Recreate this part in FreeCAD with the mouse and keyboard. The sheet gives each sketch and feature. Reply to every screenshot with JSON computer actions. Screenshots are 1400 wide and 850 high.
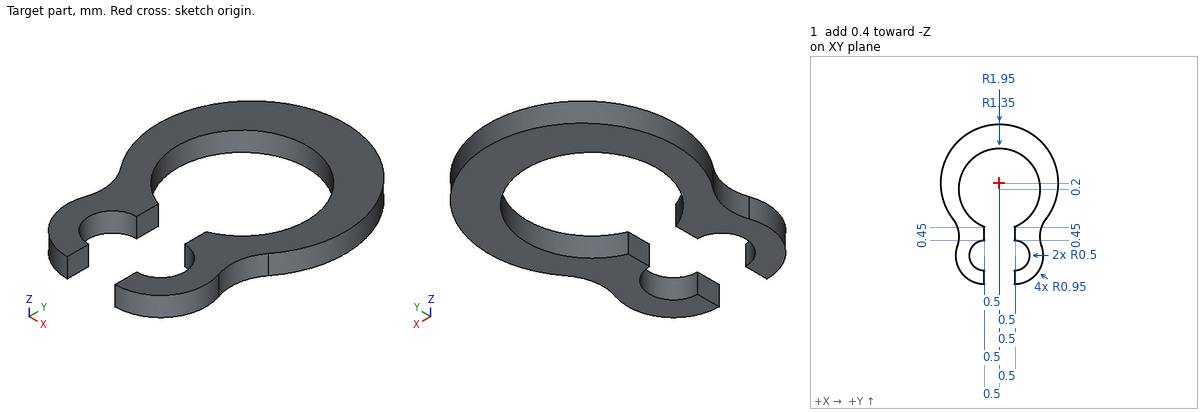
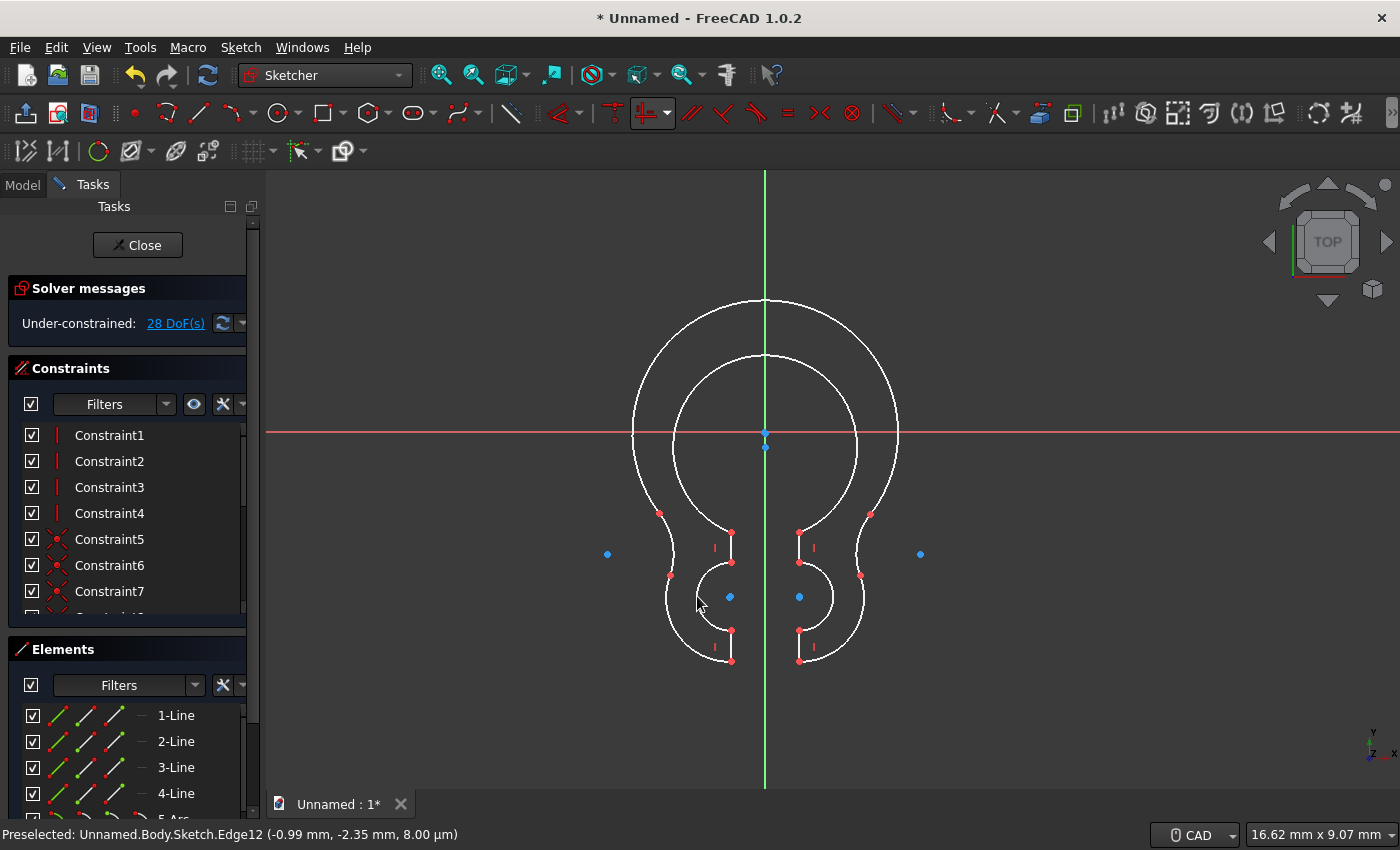
{"action": "left_click", "coordinate": [834, 652]}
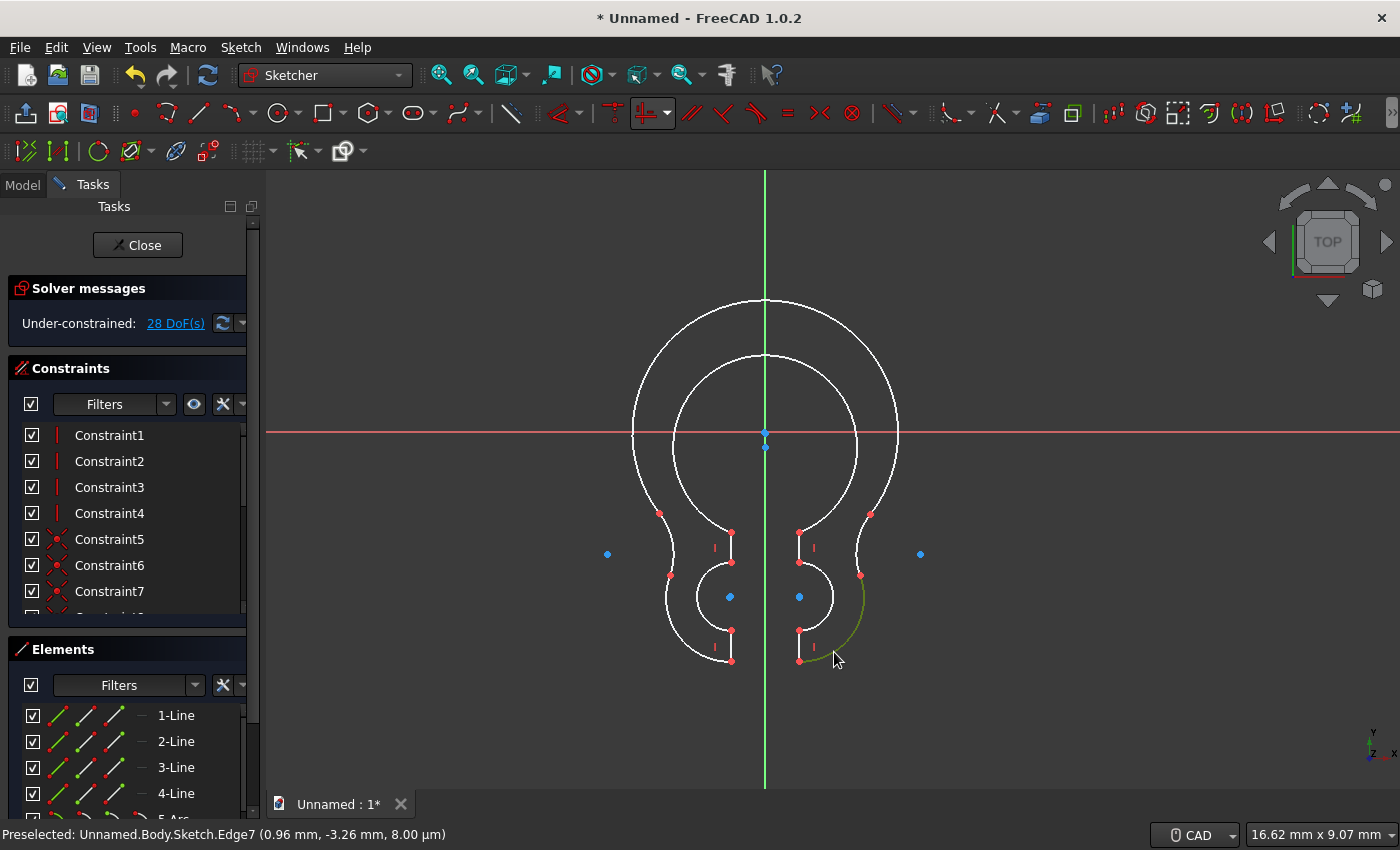
{"action": "left_click", "coordinate": [861, 532]}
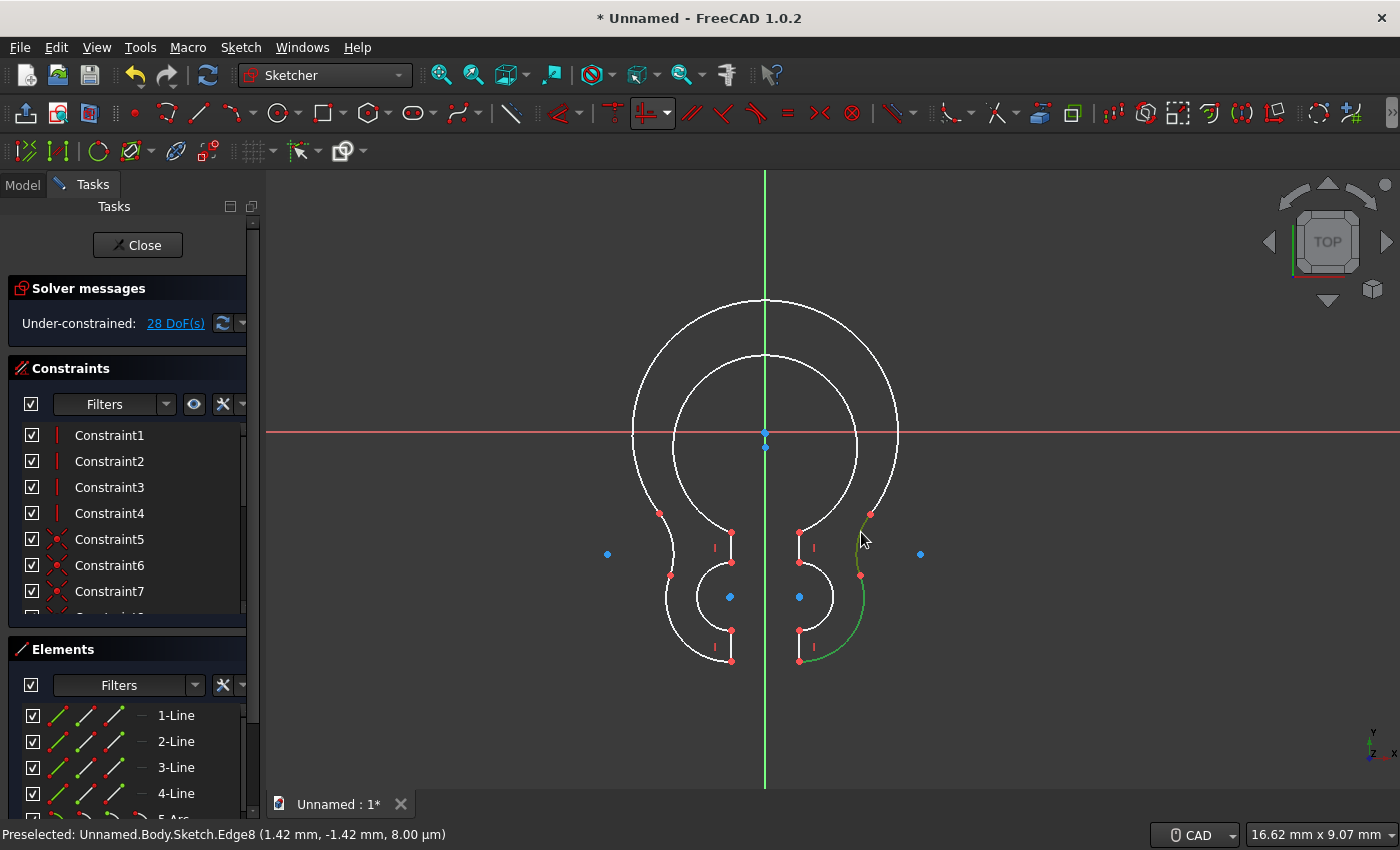
{"action": "left_click", "coordinate": [756, 114]}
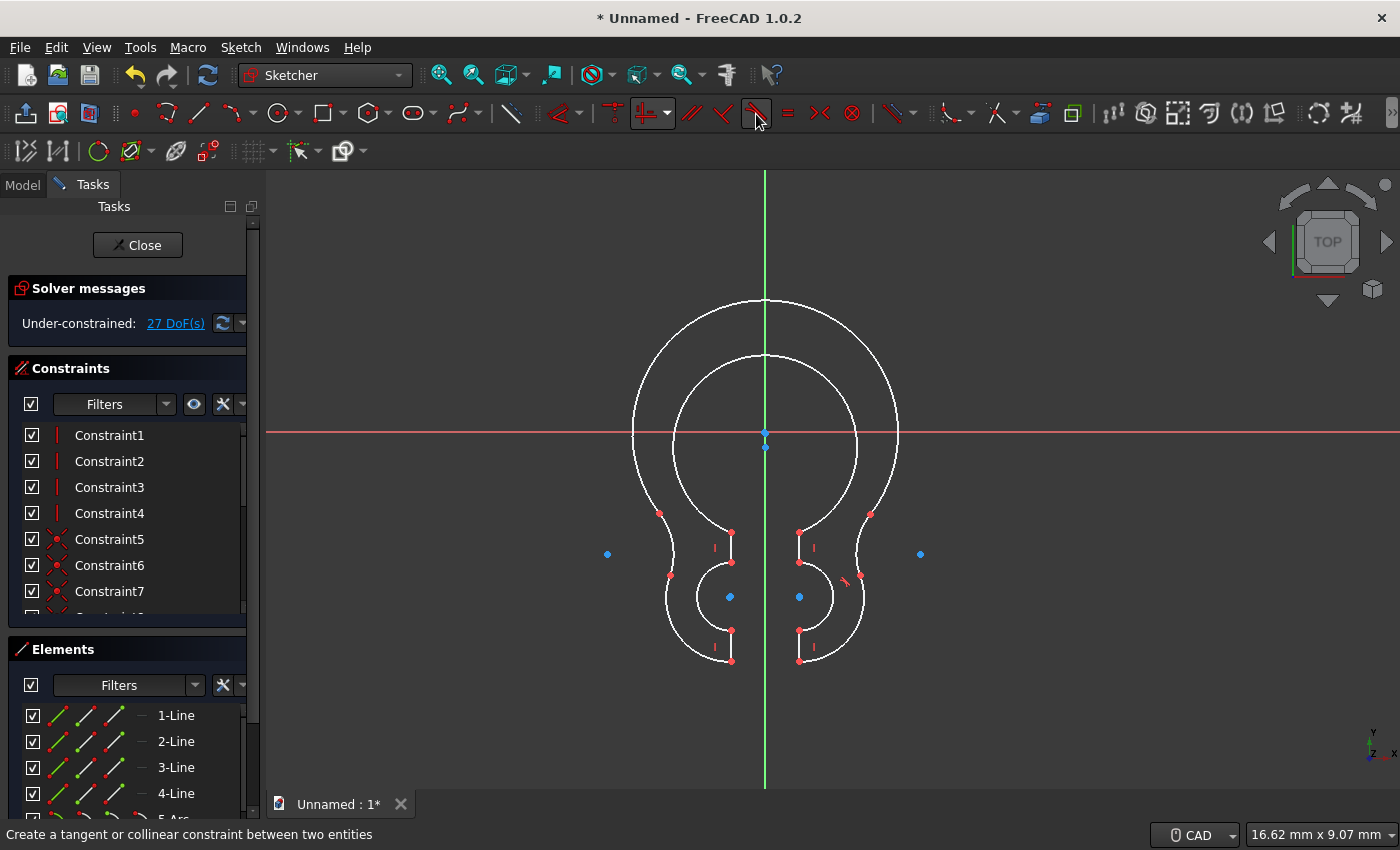
{"action": "left_click", "coordinate": [861, 532]}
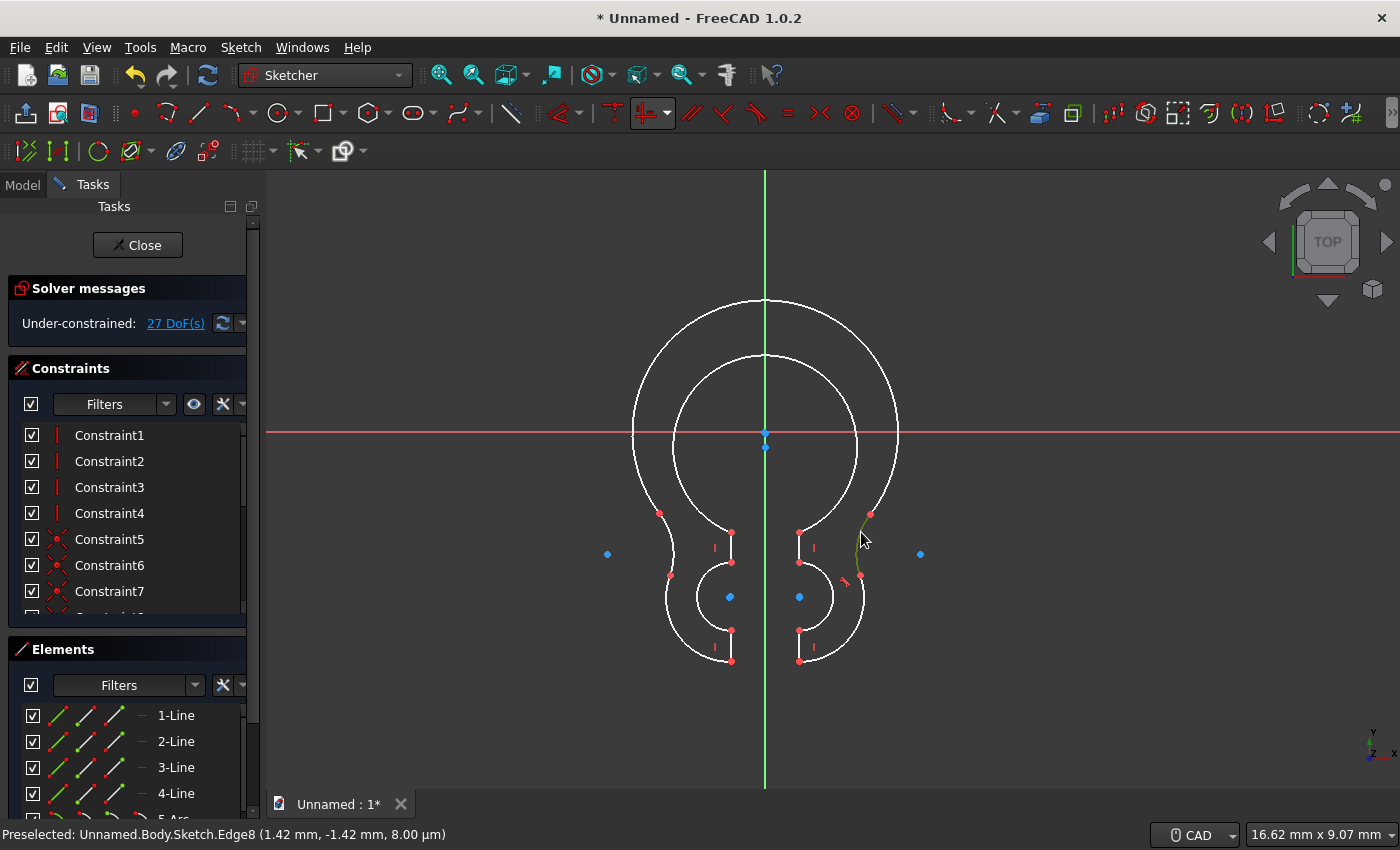
{"action": "left_click", "coordinate": [869, 350]}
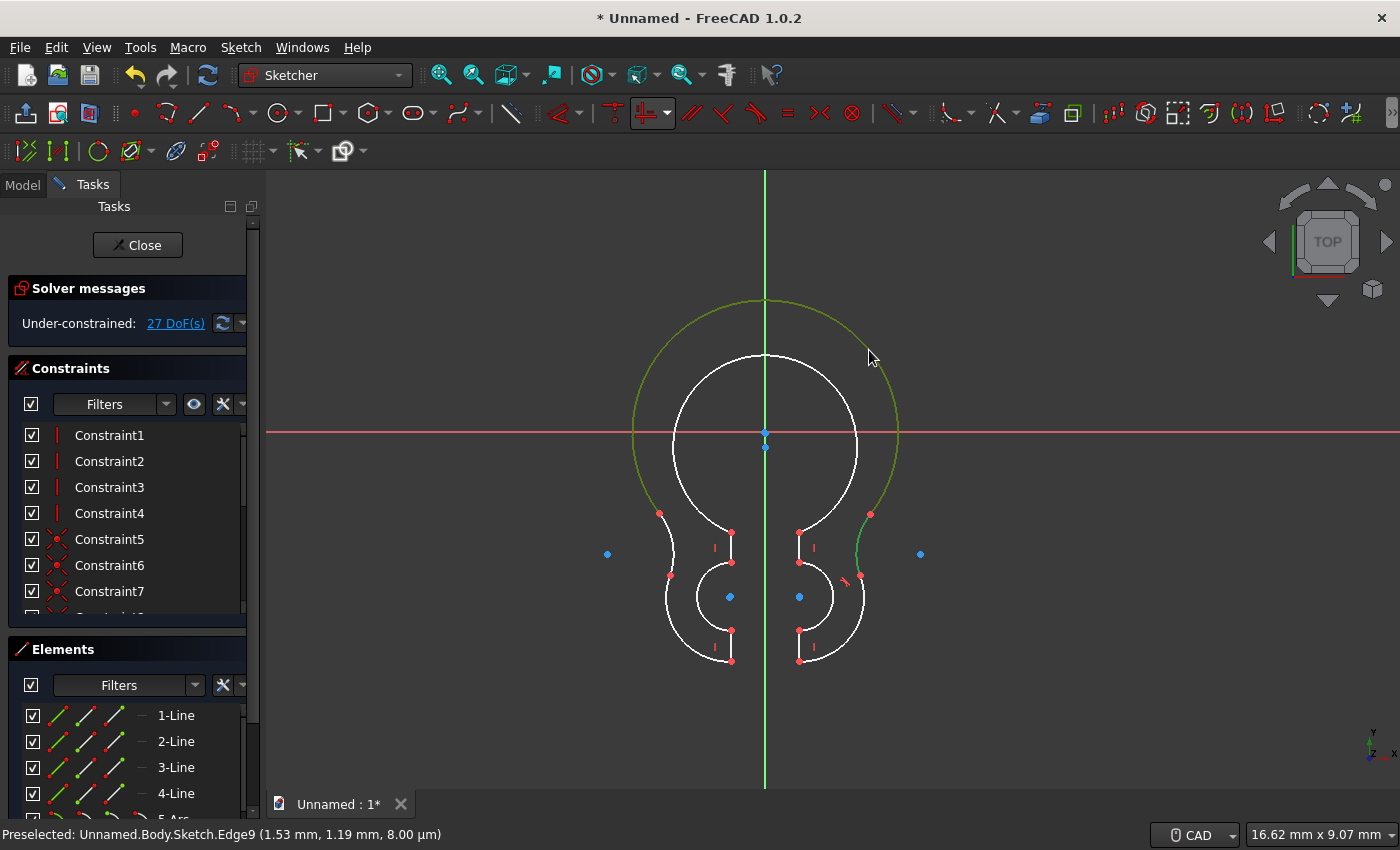
{"action": "left_click", "coordinate": [756, 114]}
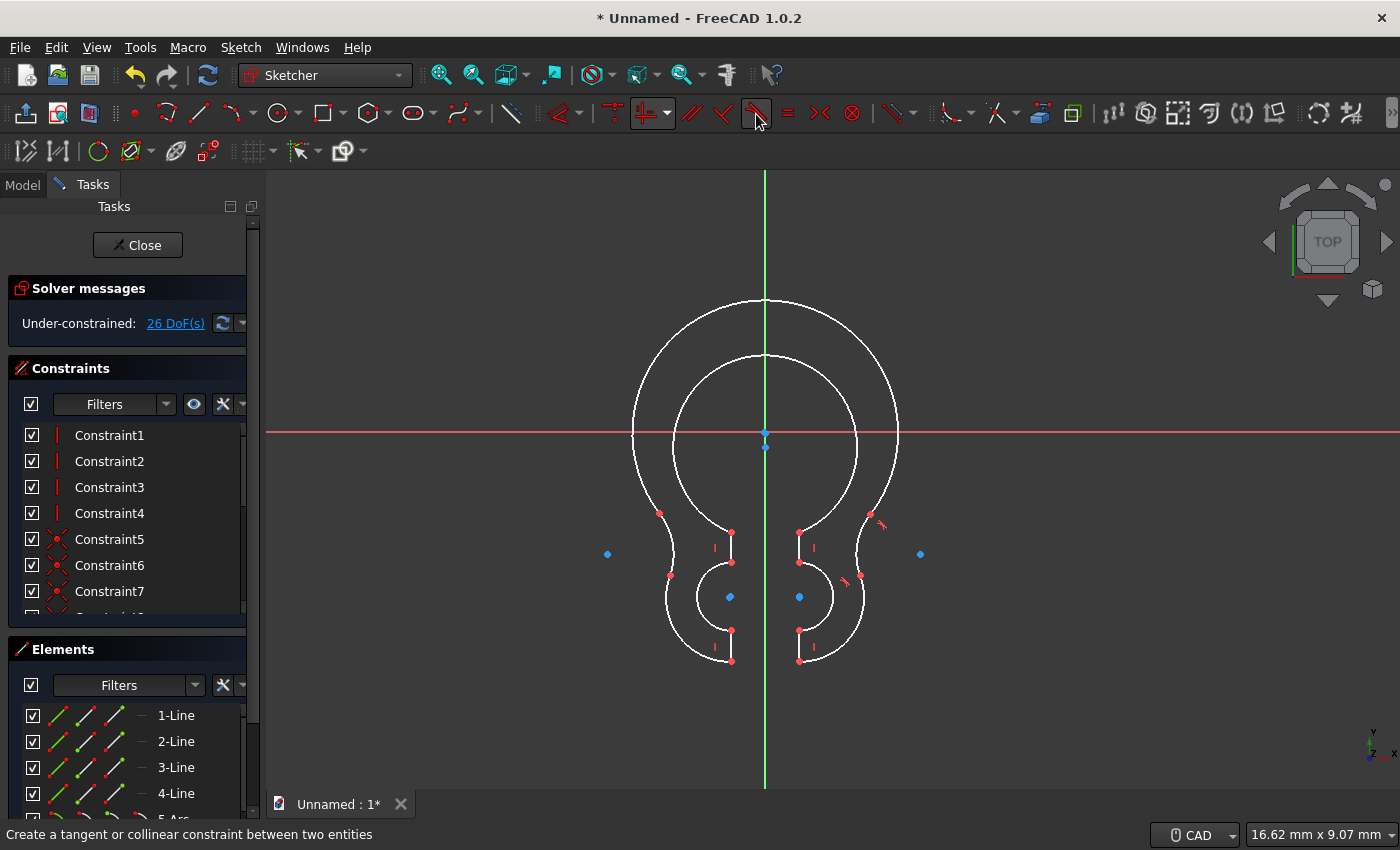
{"action": "left_click", "coordinate": [869, 350]}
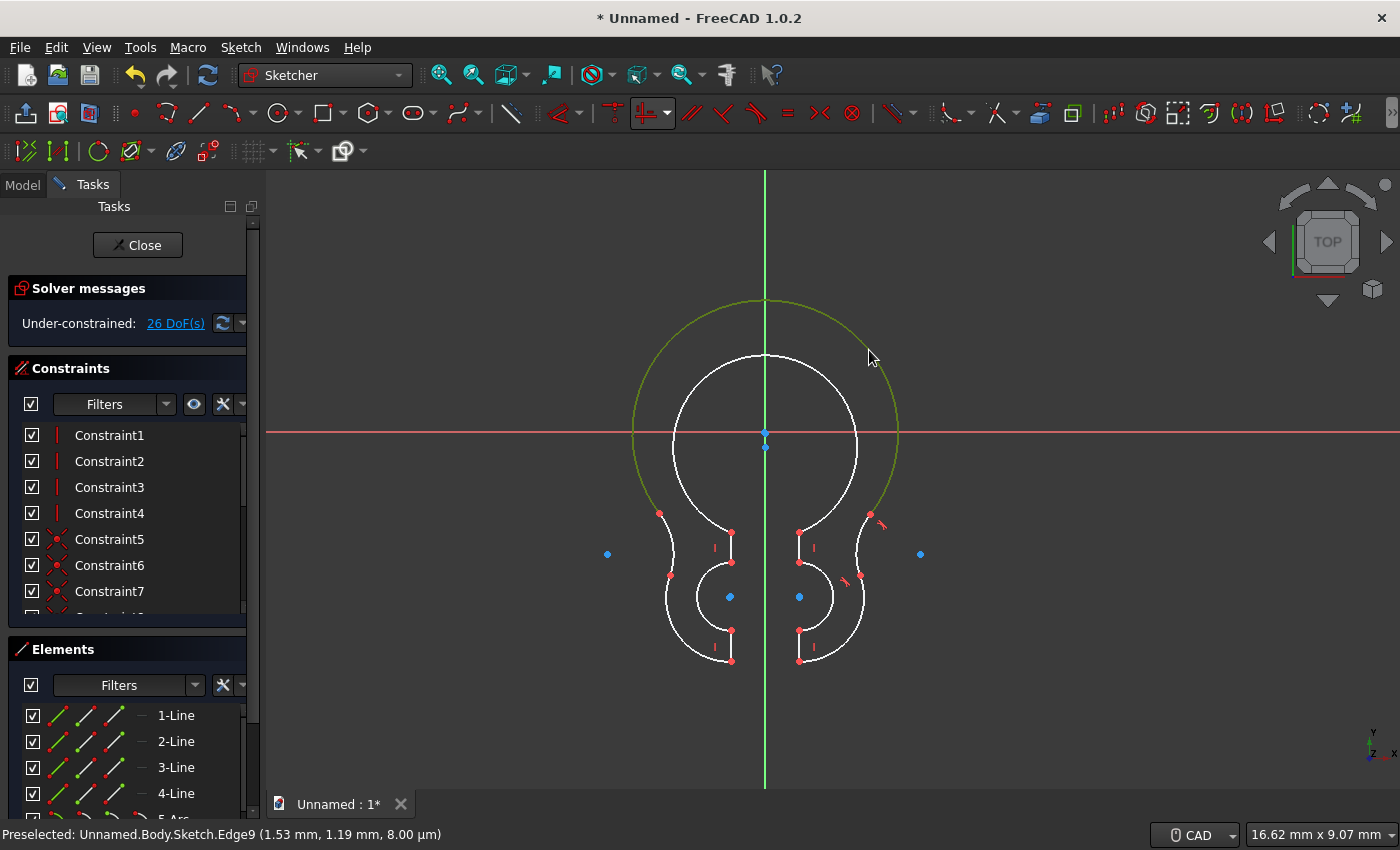
{"action": "left_click", "coordinate": [674, 557]}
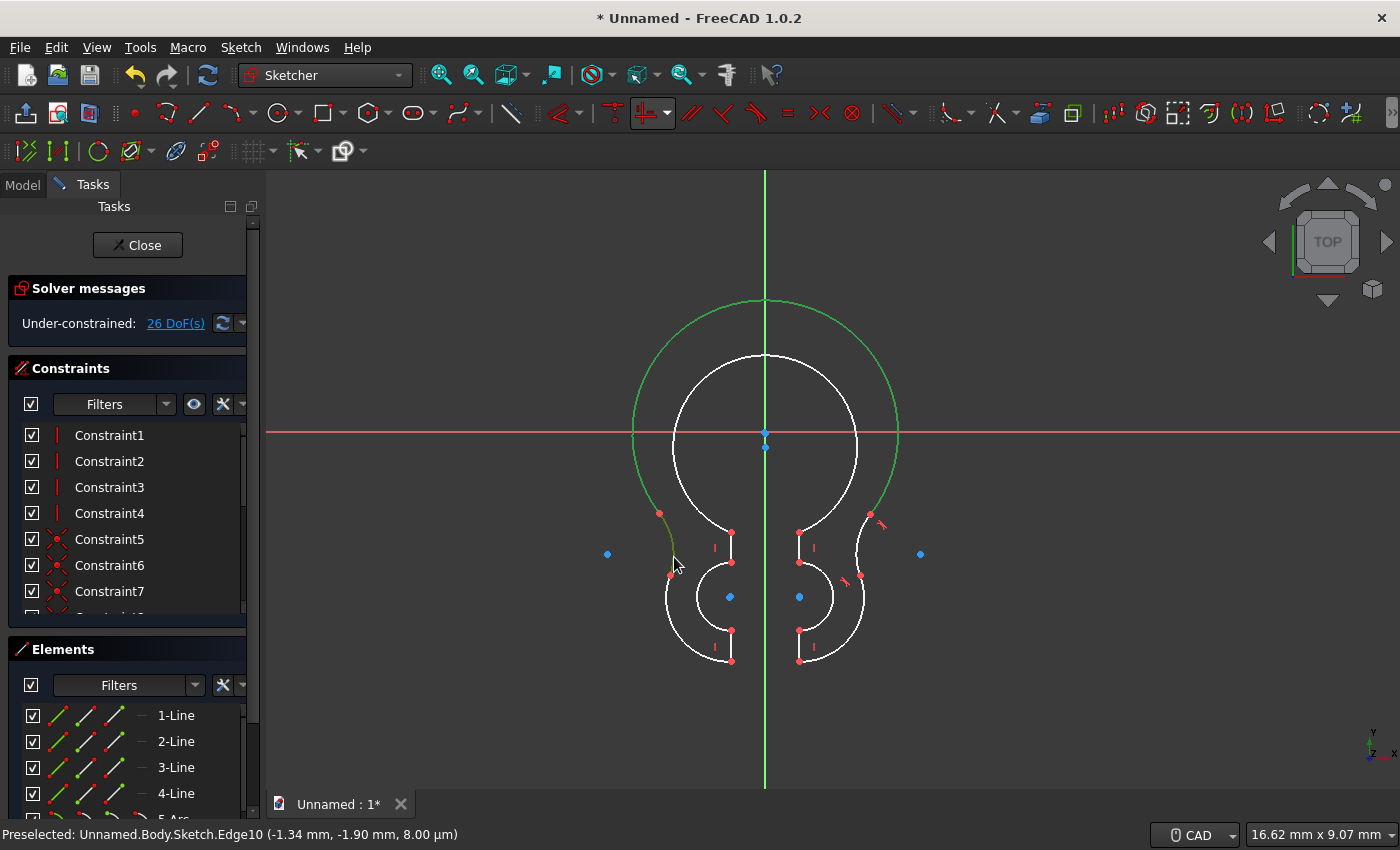
{"action": "left_click", "coordinate": [756, 114]}